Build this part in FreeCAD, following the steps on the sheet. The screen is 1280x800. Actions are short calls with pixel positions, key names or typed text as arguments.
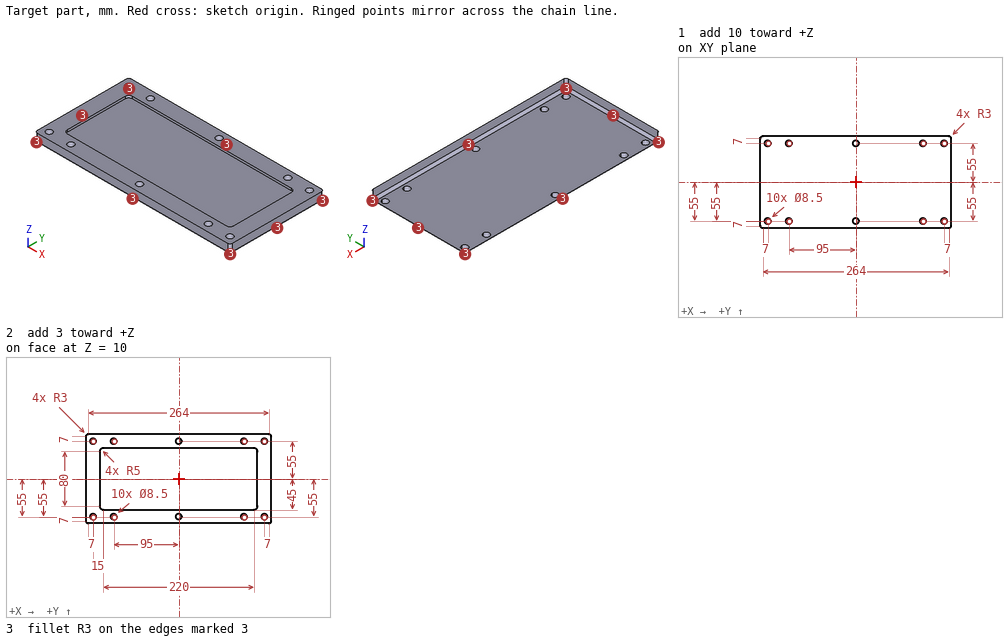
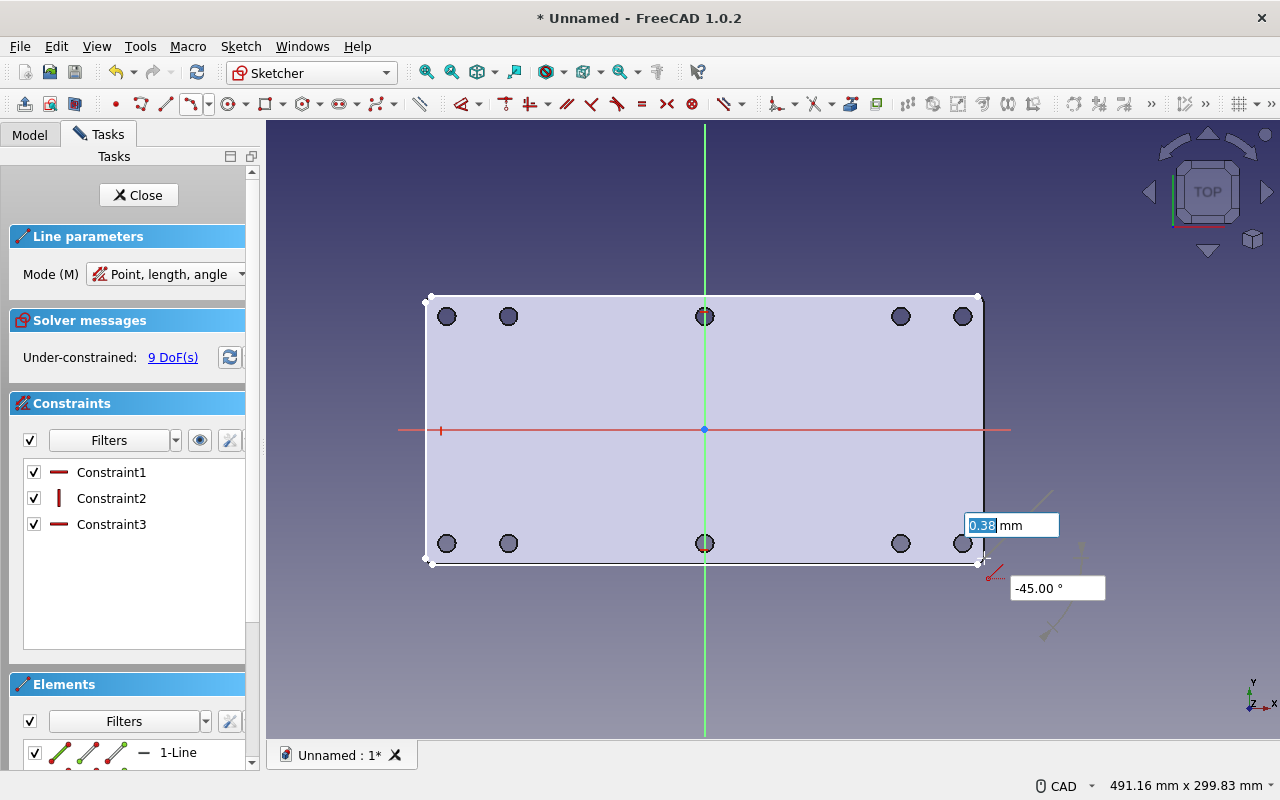
scroll(984, 302, up, 3)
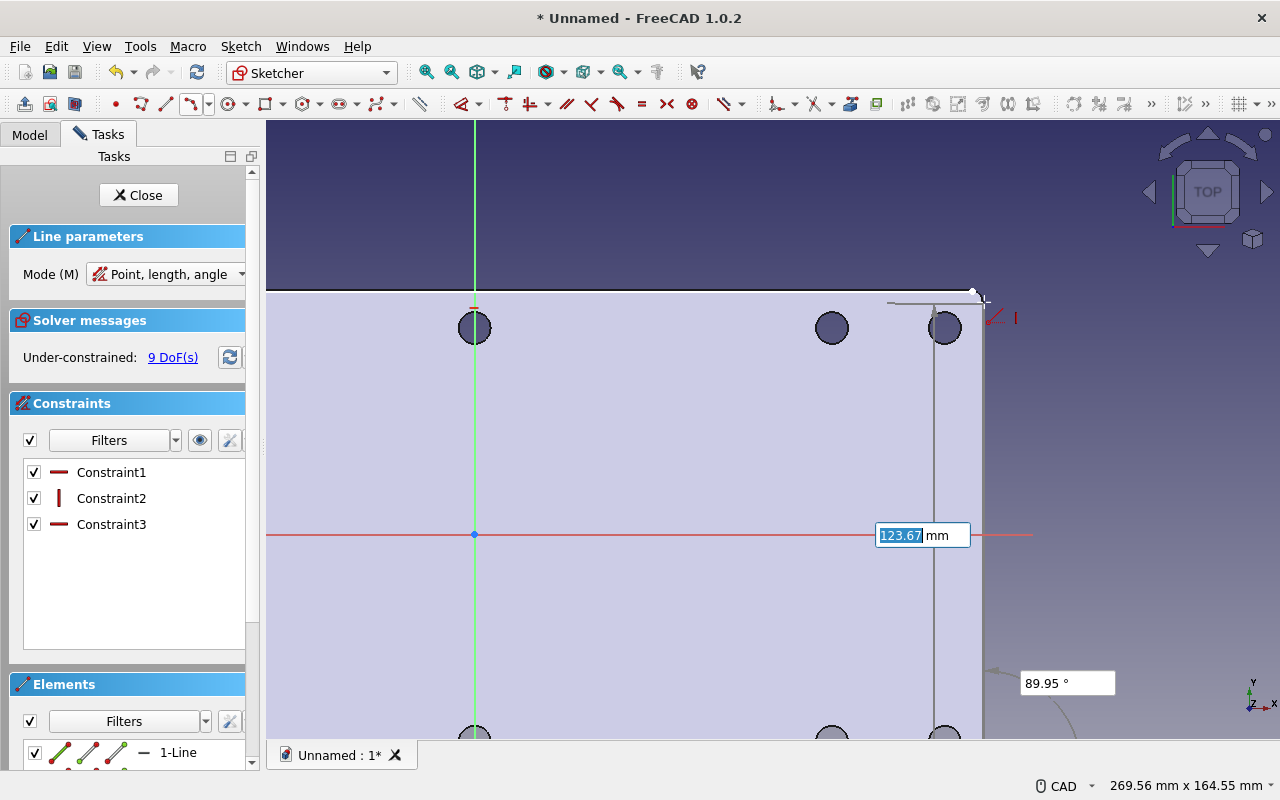
click(983, 302)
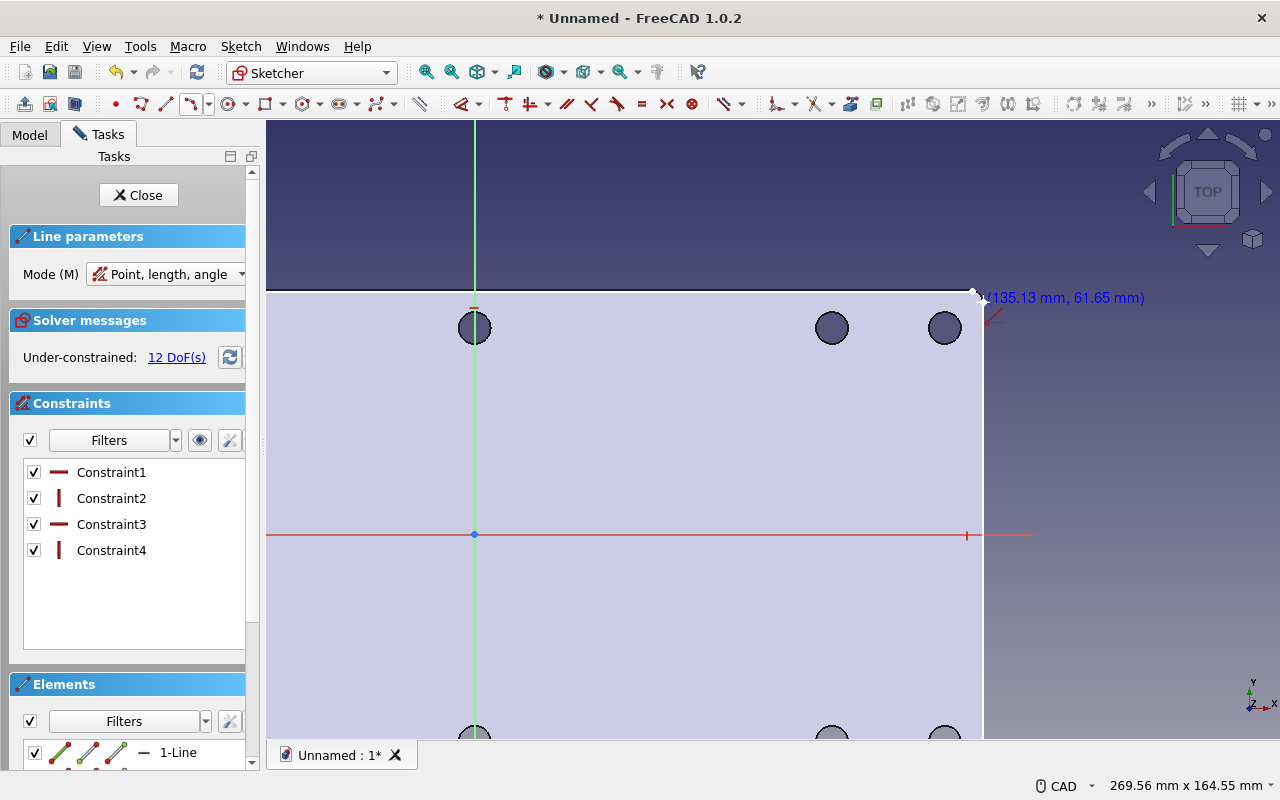
click(190, 104)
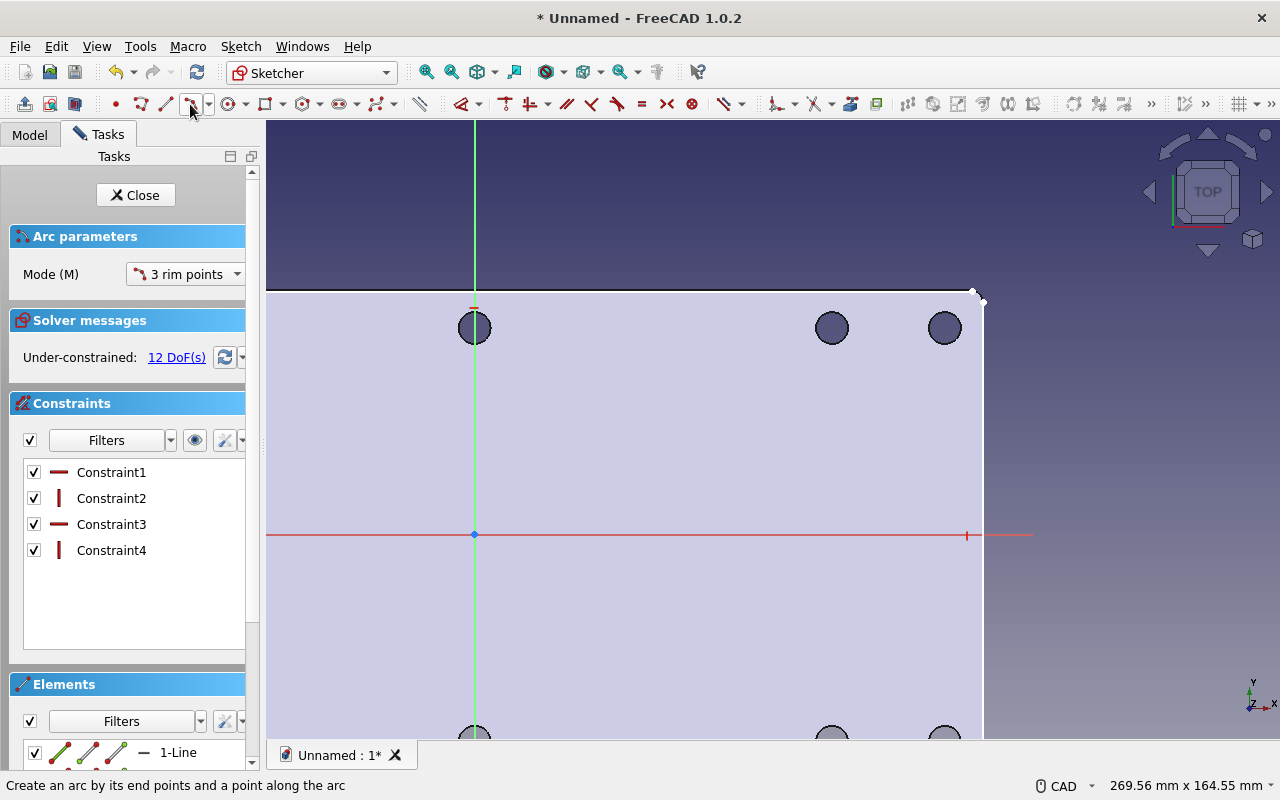
scroll(984, 301, down, 3)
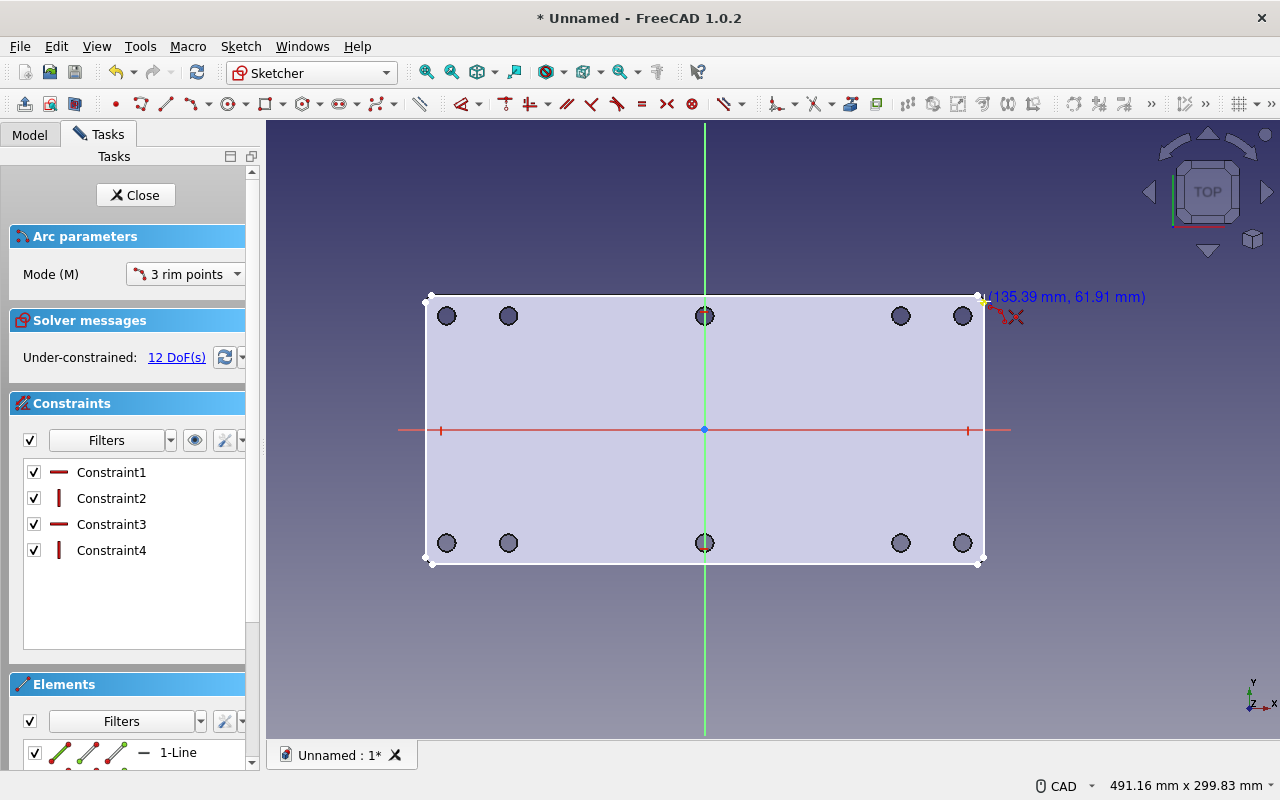
scroll(432, 295, up, 3)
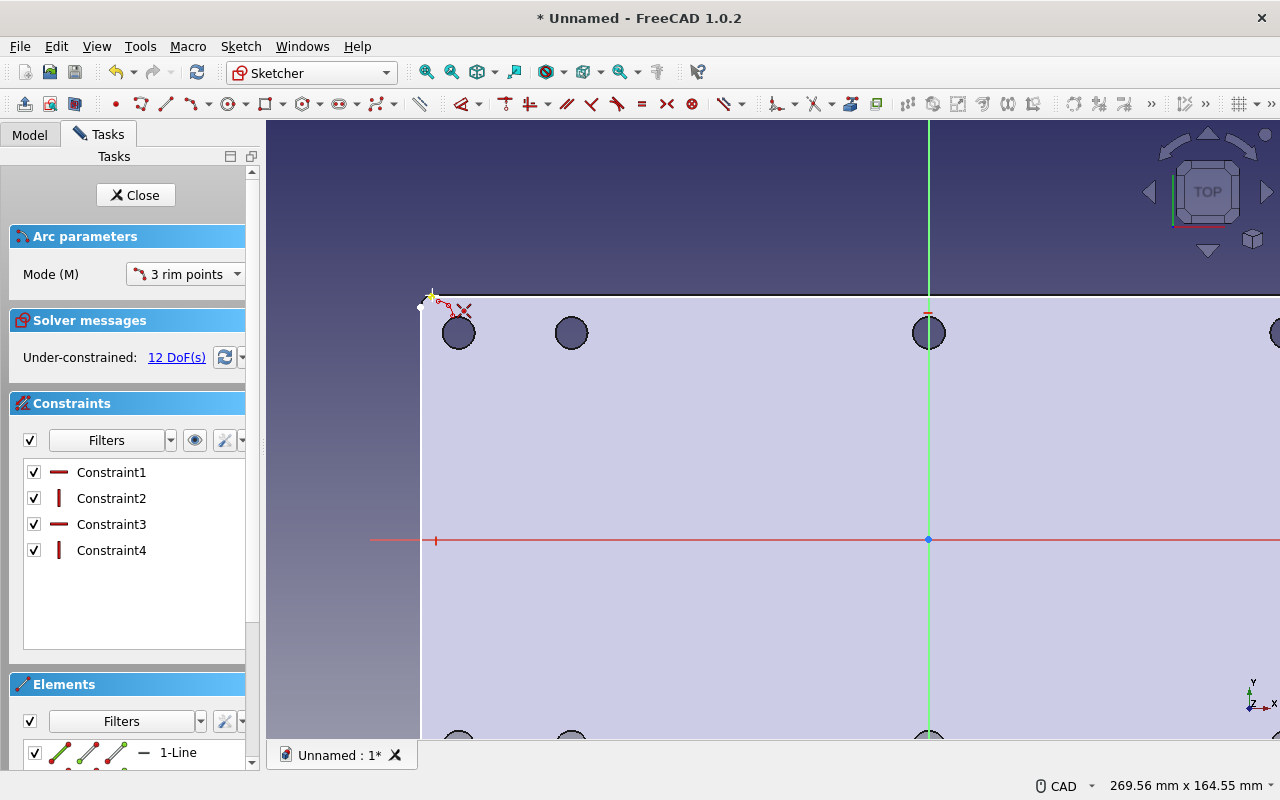
click(432, 297)
click(421, 308)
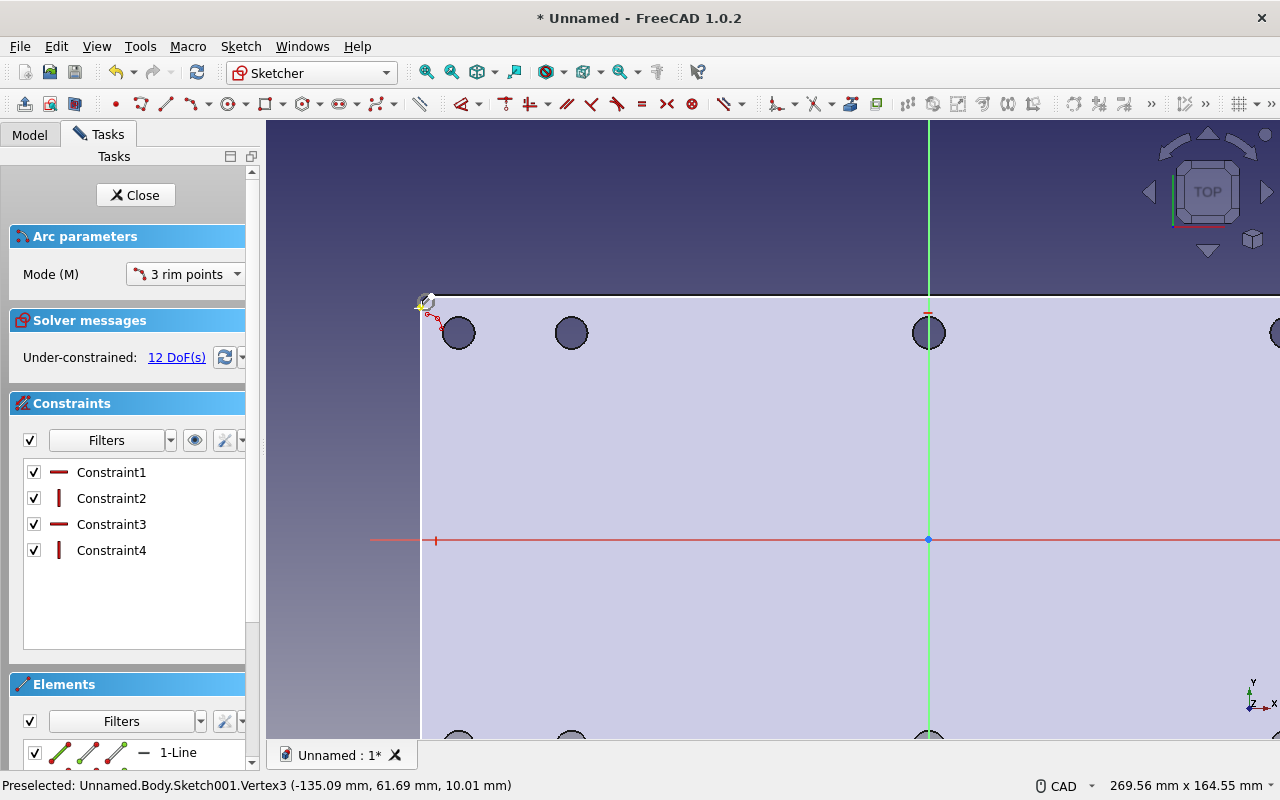
scroll(424, 299, up, 8)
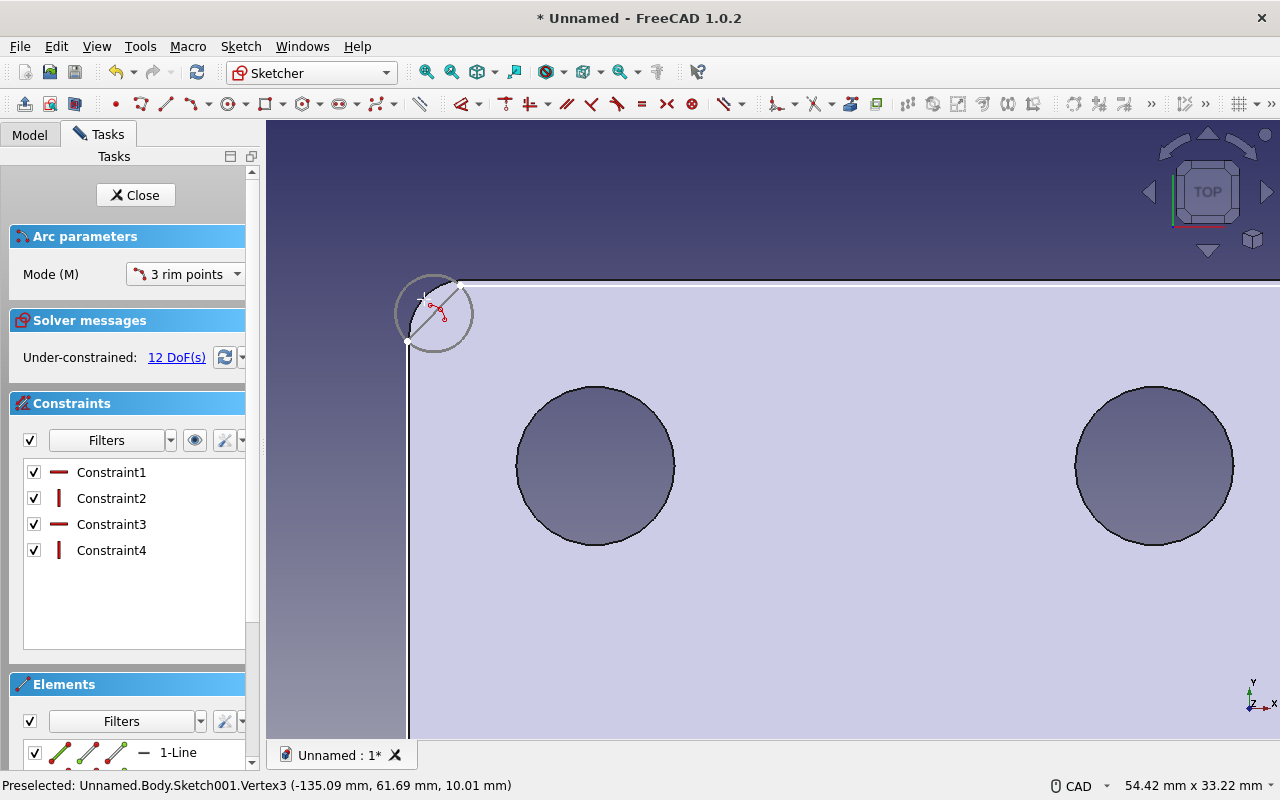
click(425, 296)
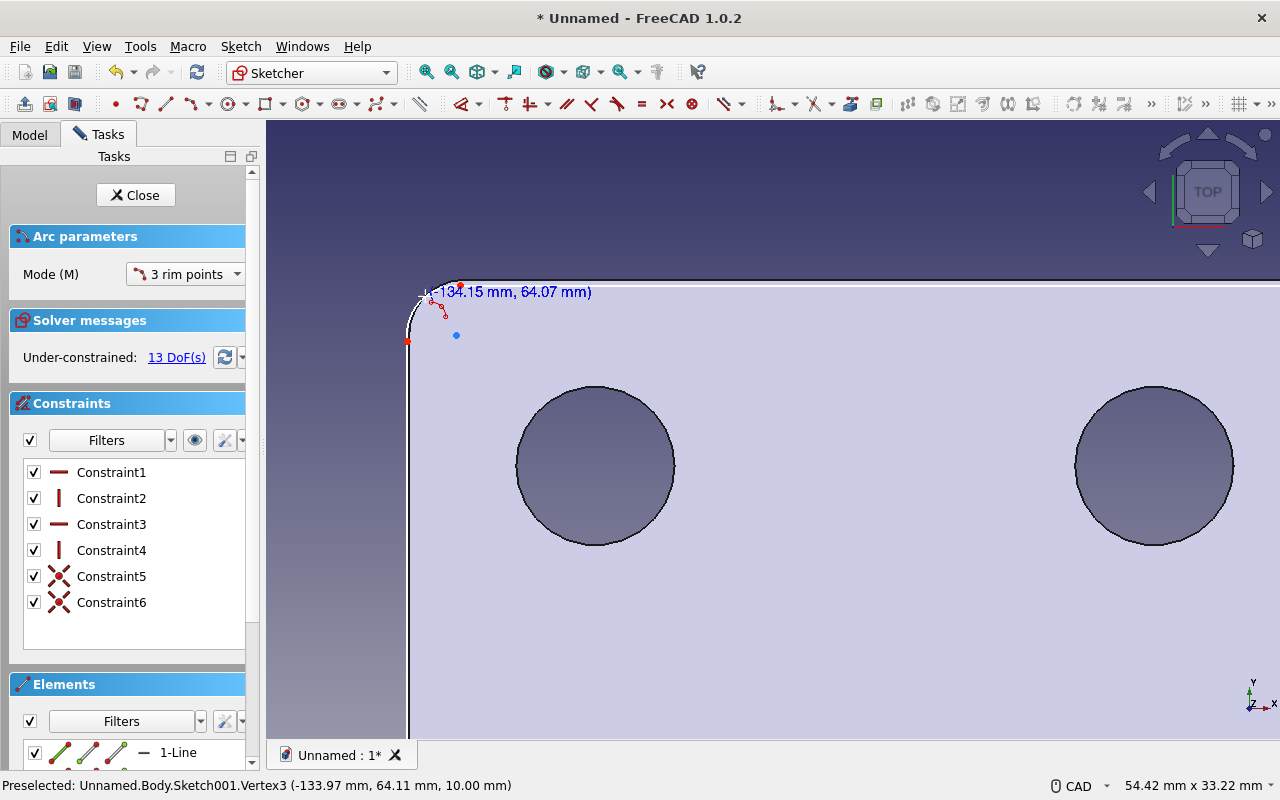
scroll(428, 297, down, 11)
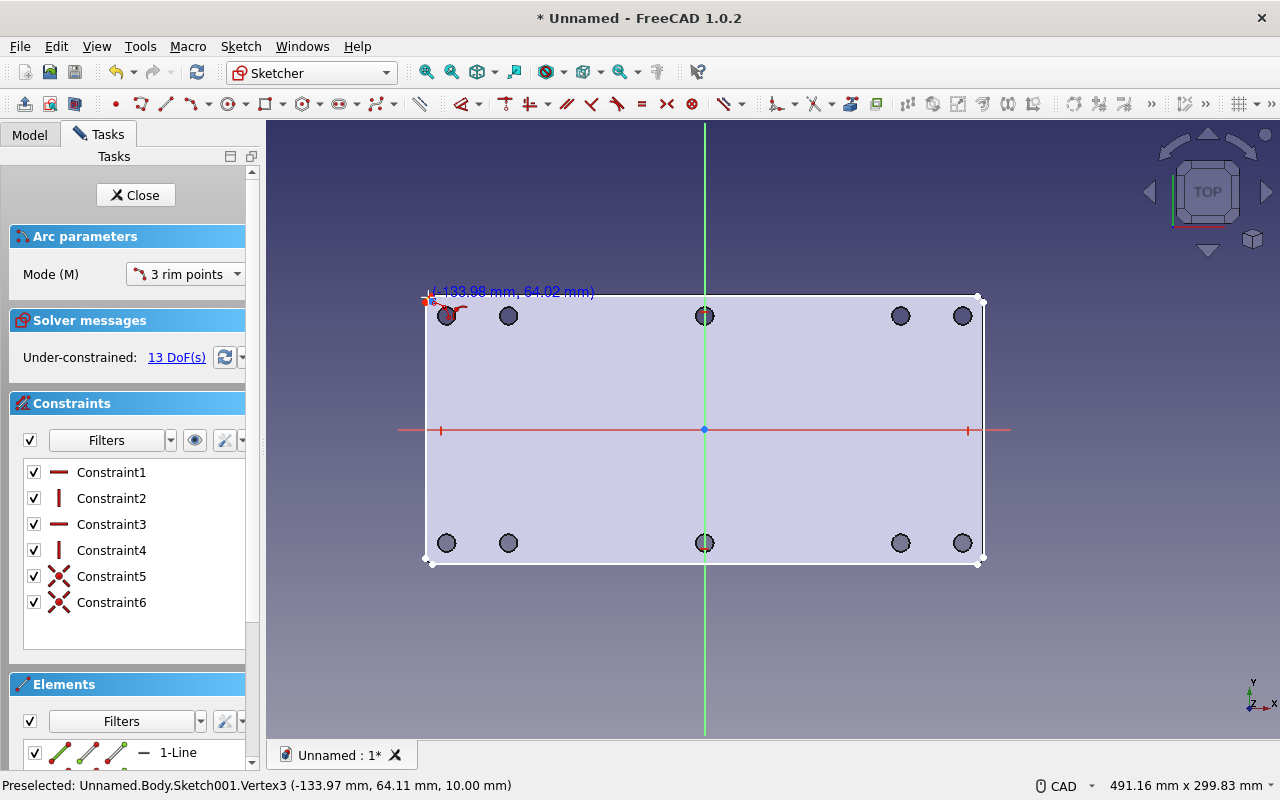
scroll(426, 558, up, 3)